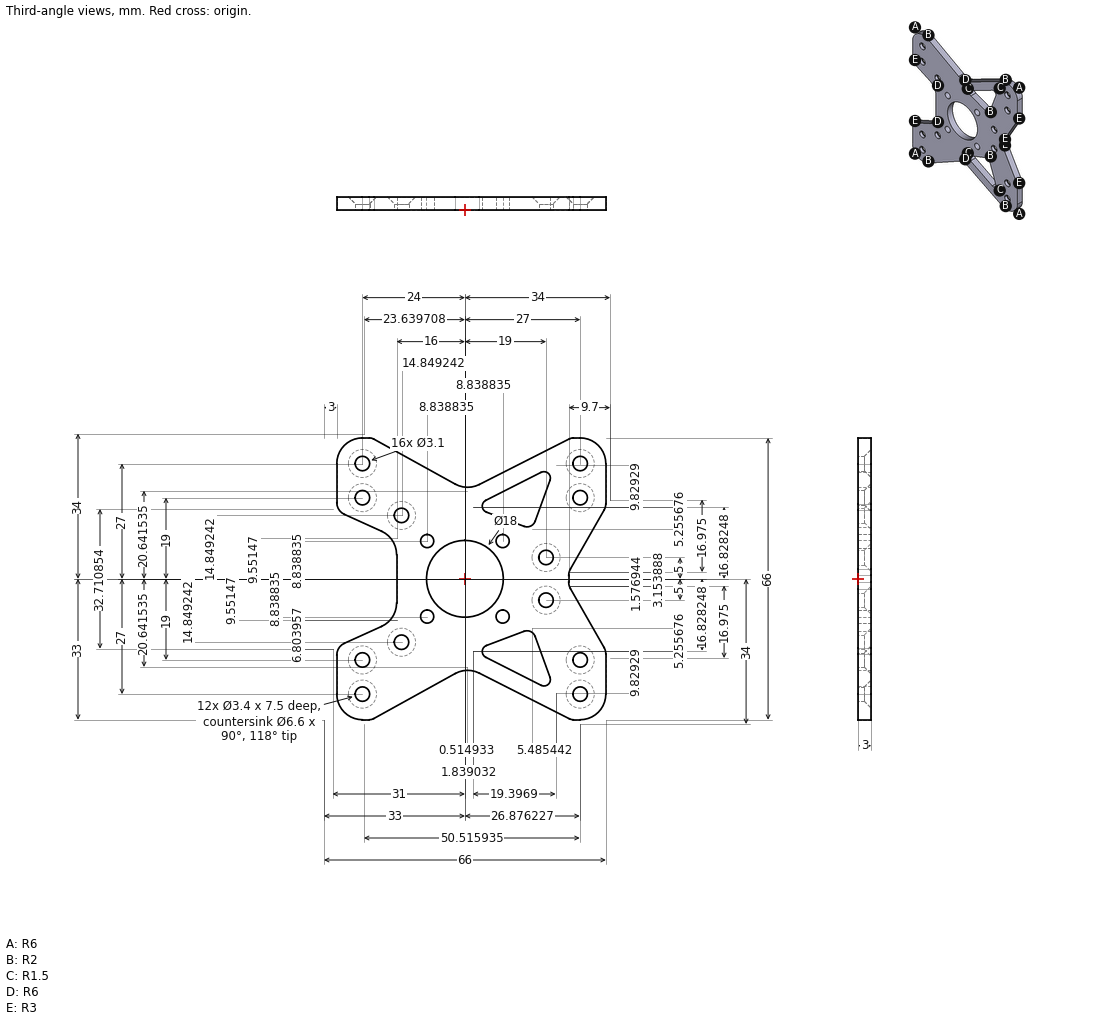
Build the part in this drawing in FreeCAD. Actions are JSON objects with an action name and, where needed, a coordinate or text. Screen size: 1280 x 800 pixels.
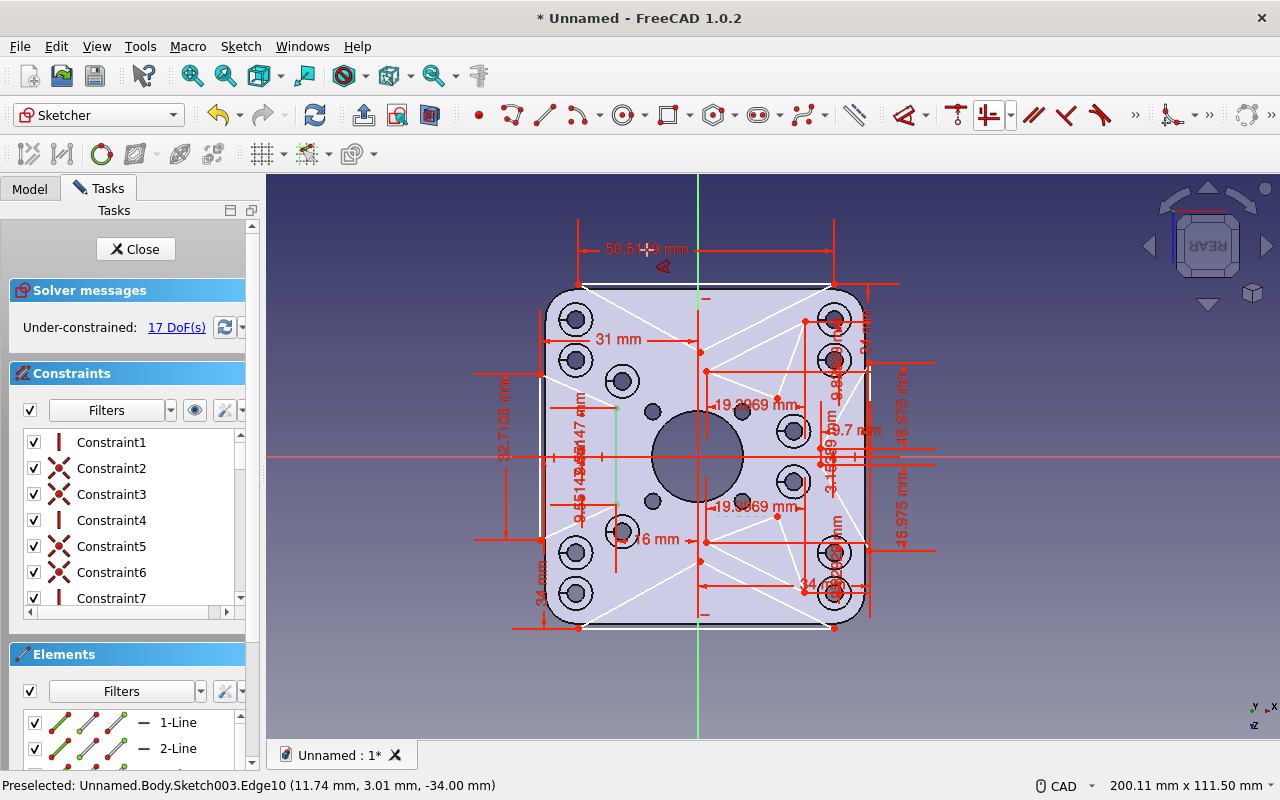
{"action": "left_click", "coordinate": [655, 629]}
{"action": "left_click", "coordinate": [647, 663]}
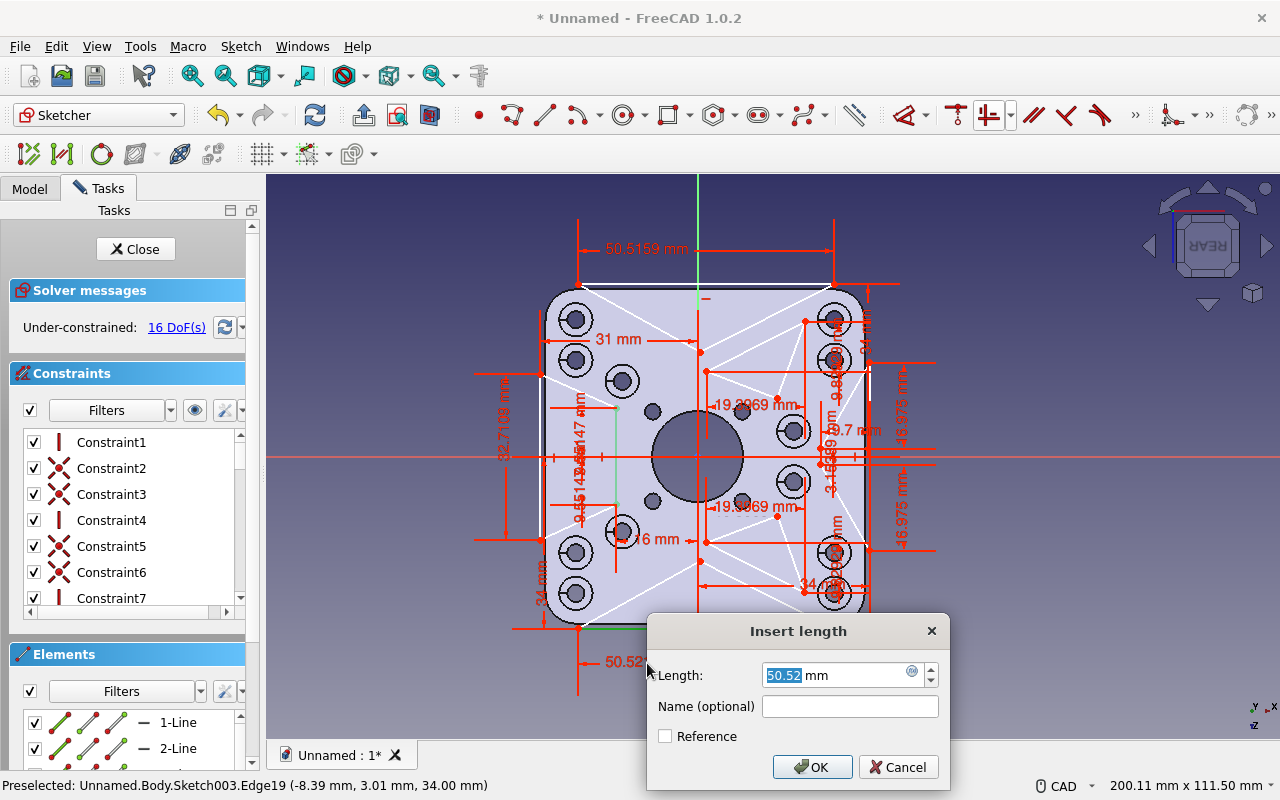
{"action": "type", "text": "50.515935"}
{"action": "key", "text": "Return"}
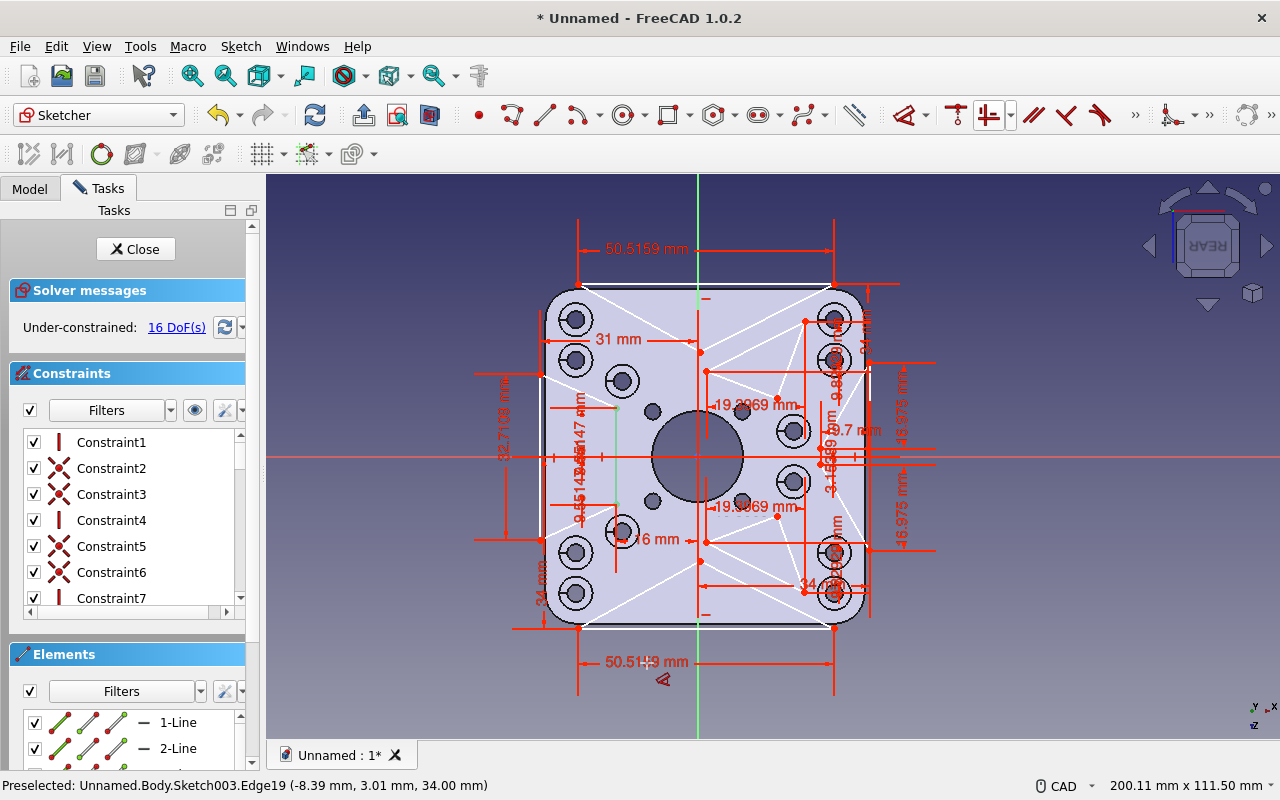
{"action": "scroll", "coordinate": [821, 449], "scroll_direction": "up", "scroll_amount": 9}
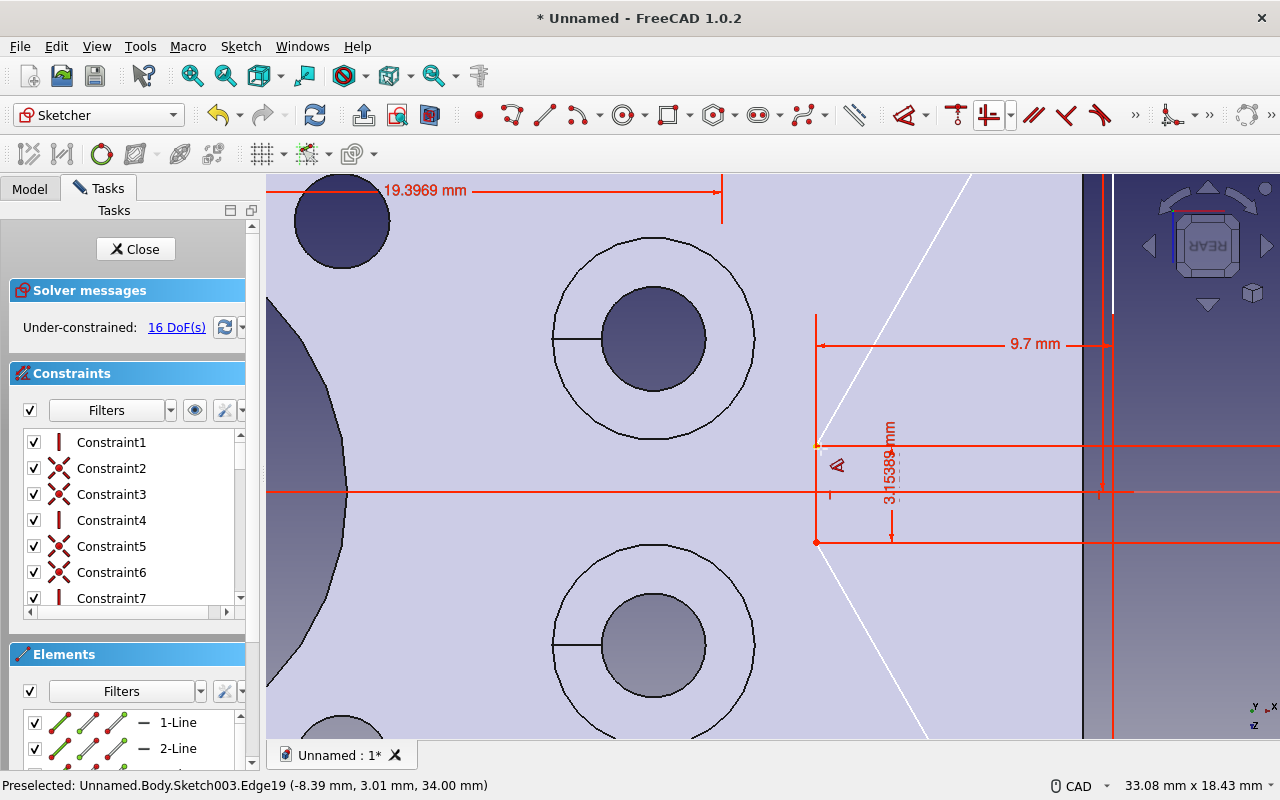
{"action": "left_click", "coordinate": [816, 446]}
{"action": "left_click", "coordinate": [970, 469]}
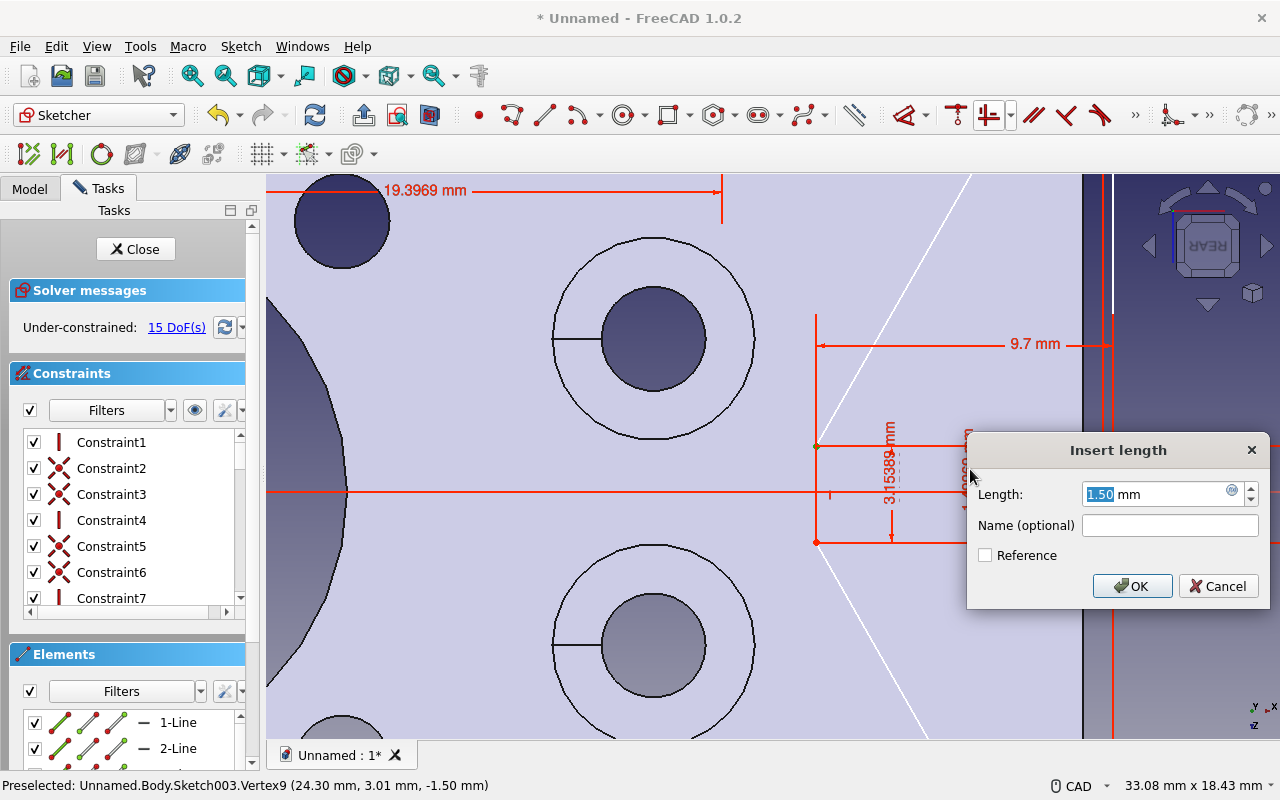
{"action": "type", "text": "1.576944"}
{"action": "key", "text": "Return"}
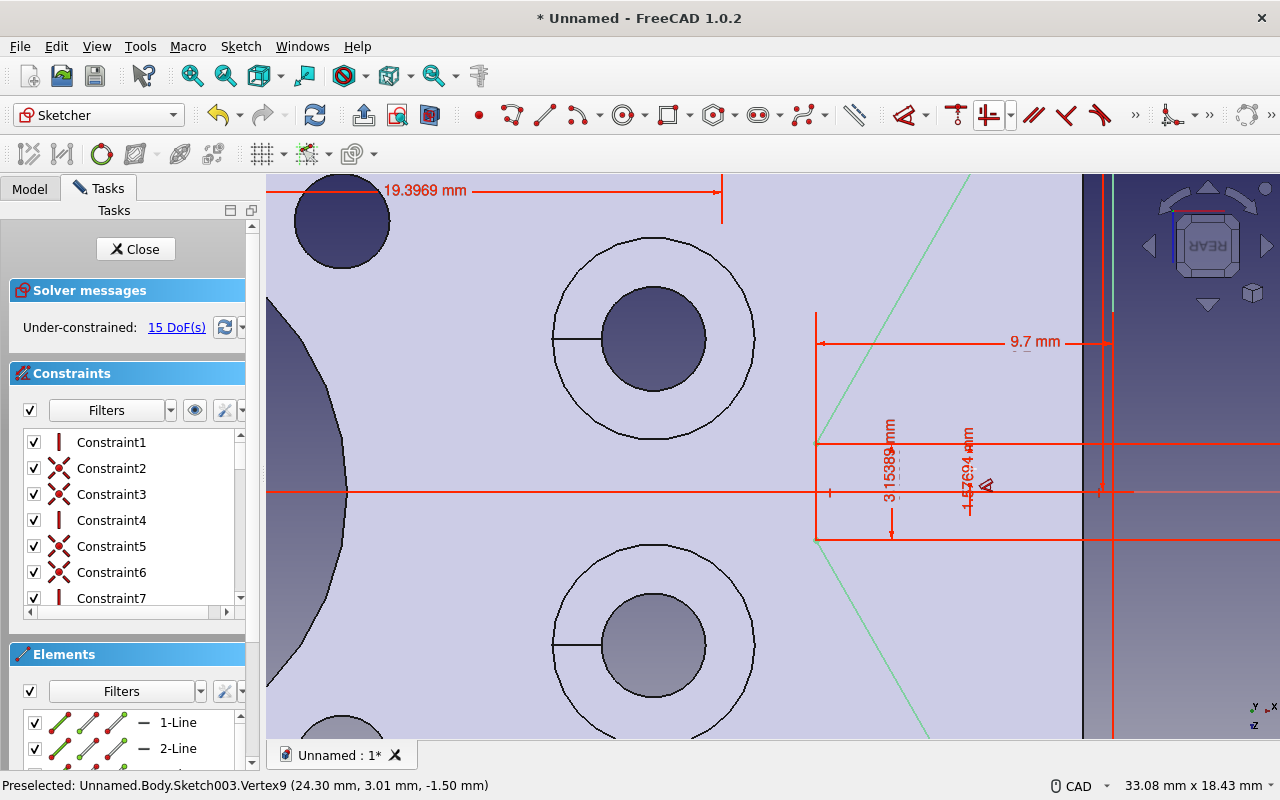
{"action": "scroll", "coordinate": [821, 449], "scroll_direction": "down", "scroll_amount": 9}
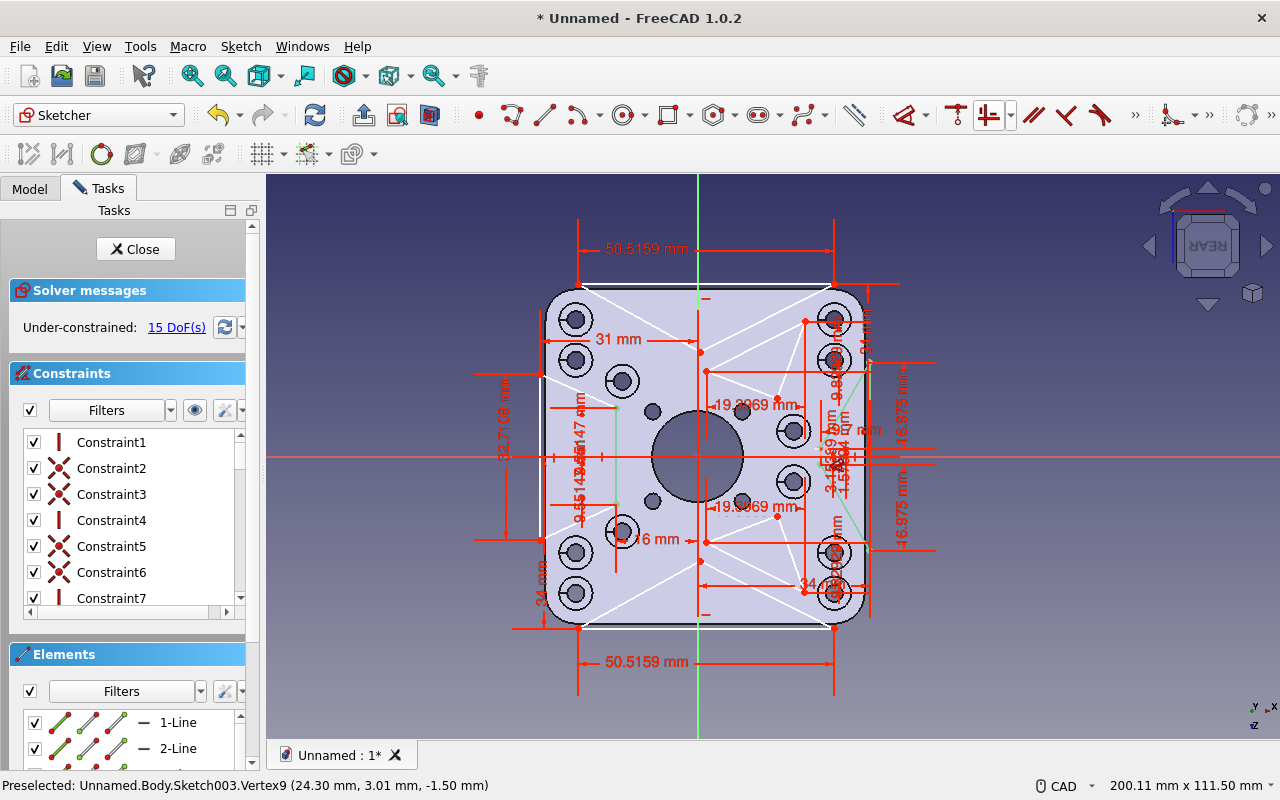
{"action": "scroll", "coordinate": [700, 352], "scroll_direction": "up", "scroll_amount": 14}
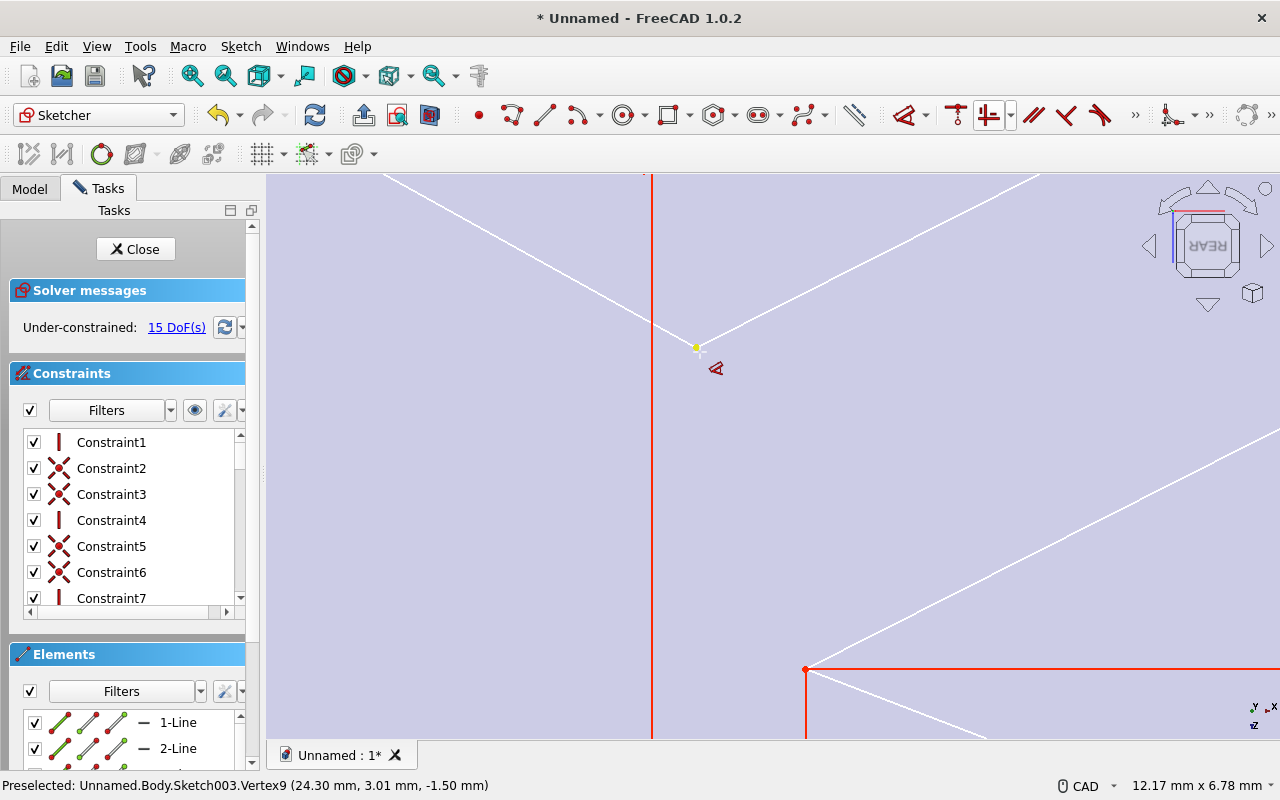
{"action": "left_click", "coordinate": [696, 348]}
{"action": "left_click", "coordinate": [674, 314]}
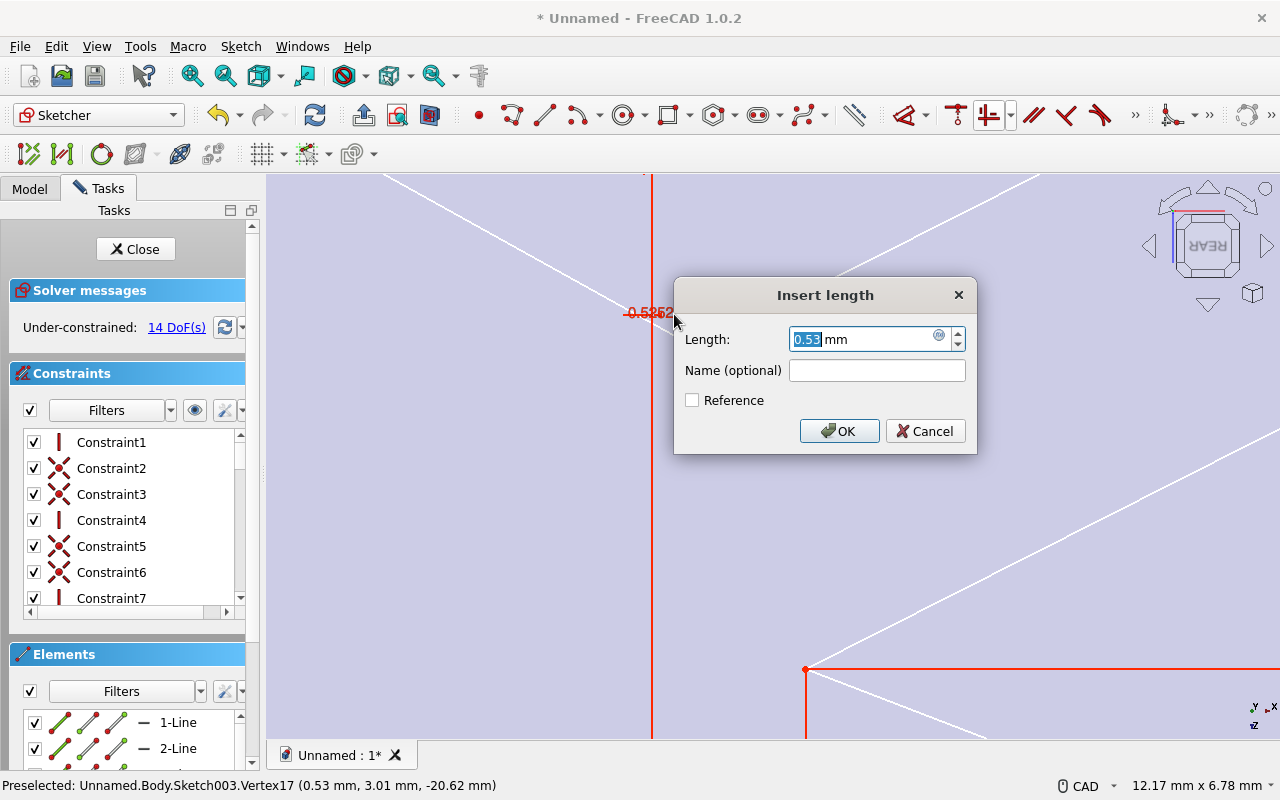
{"action": "type", "text": "0.514933"}
{"action": "key", "text": "Return"}